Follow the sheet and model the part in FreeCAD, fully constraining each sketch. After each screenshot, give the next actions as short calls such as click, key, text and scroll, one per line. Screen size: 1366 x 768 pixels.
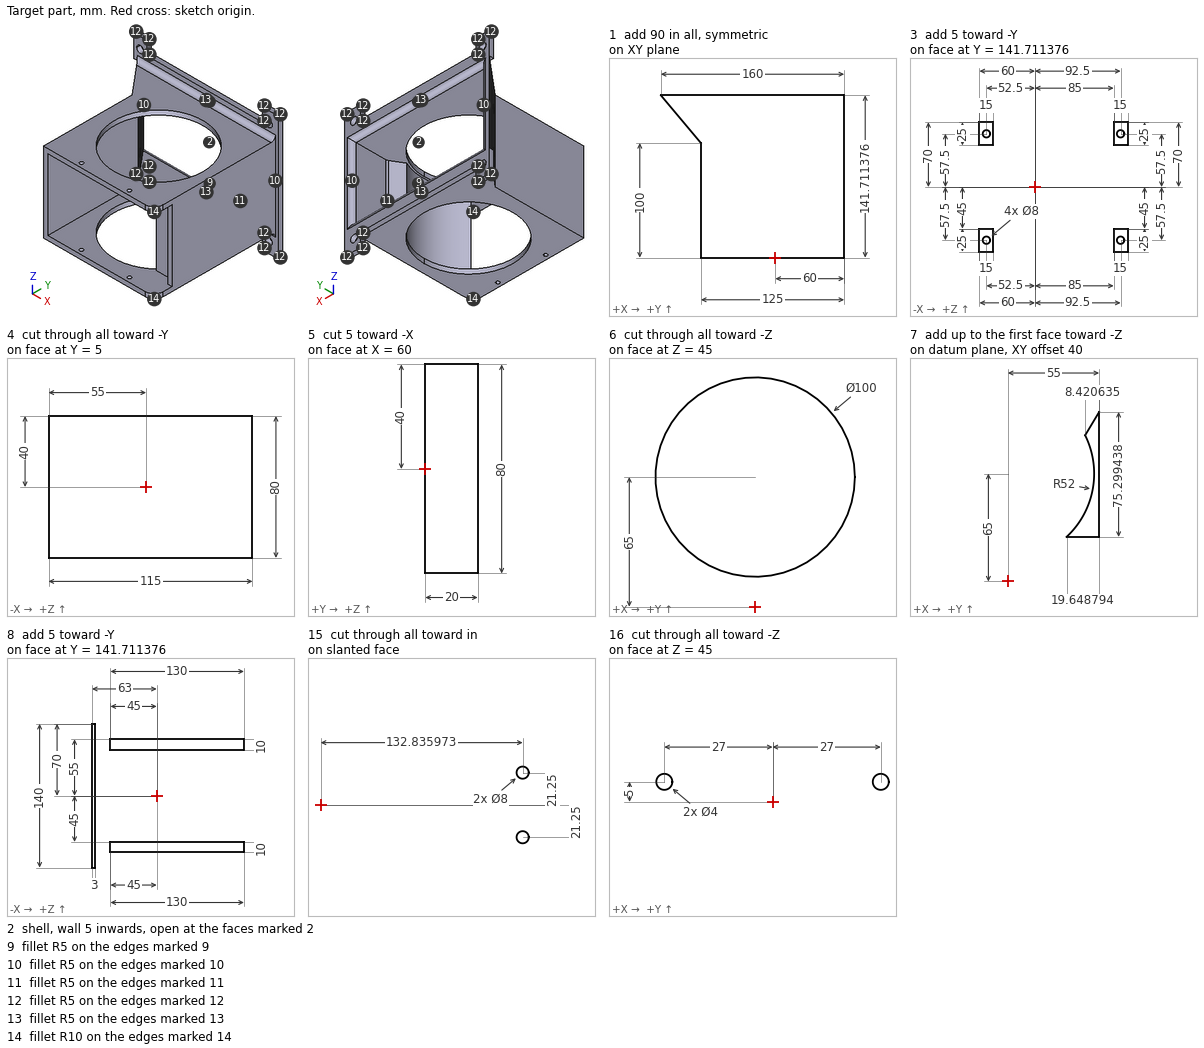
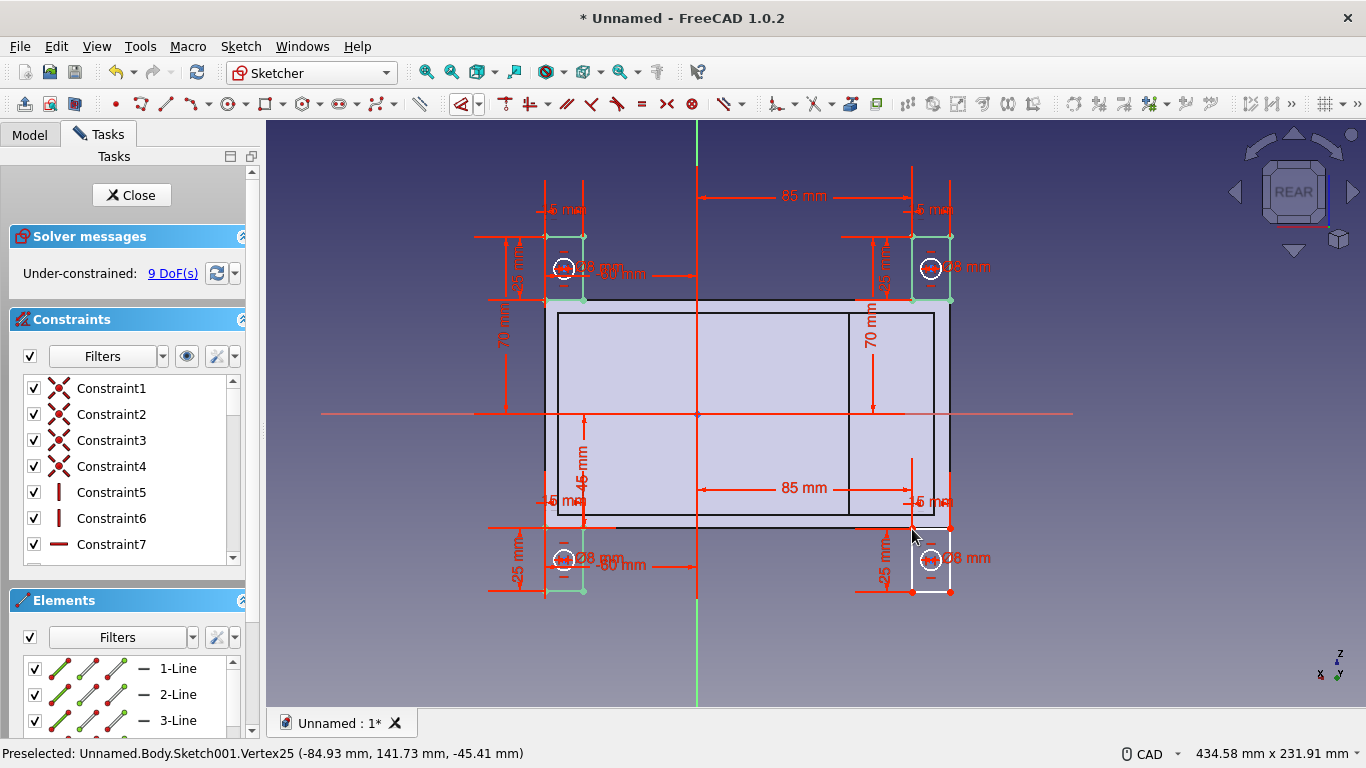
click(912, 529)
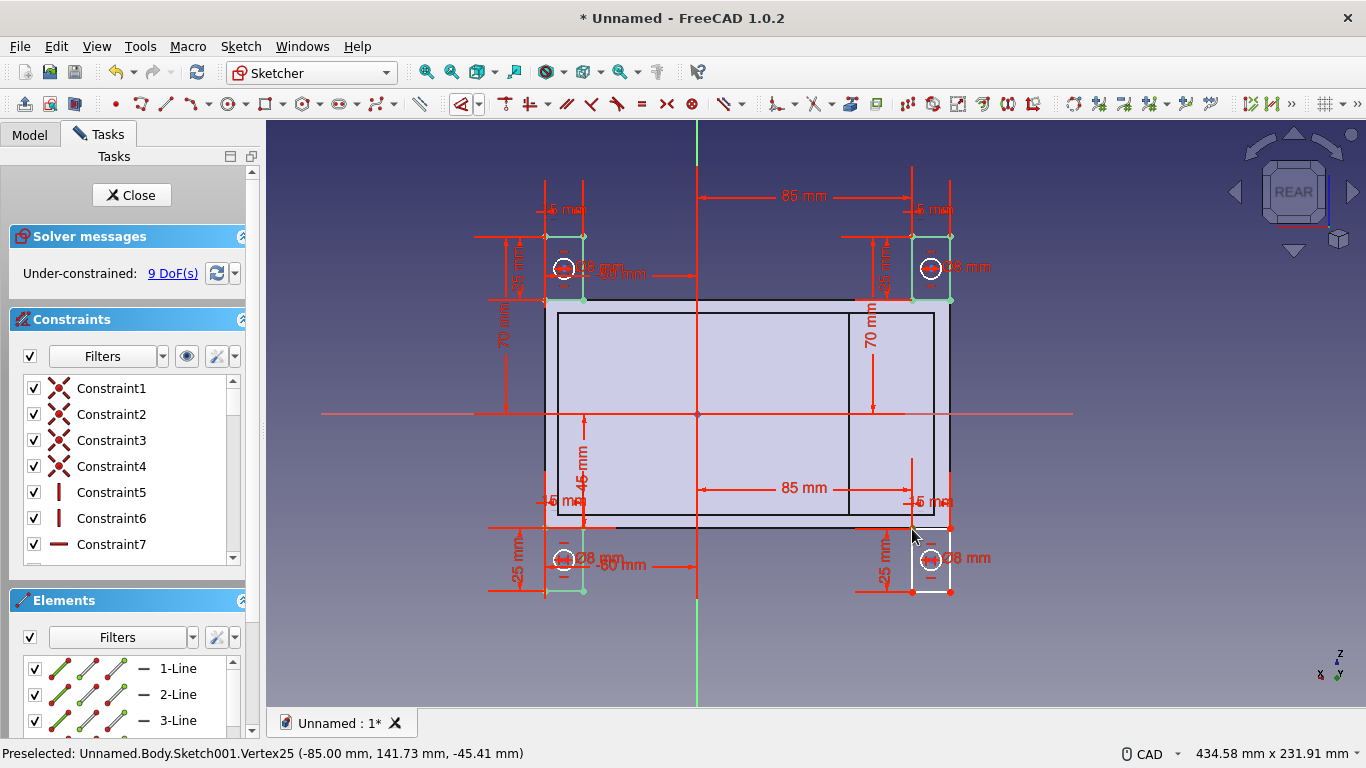
click(478, 104)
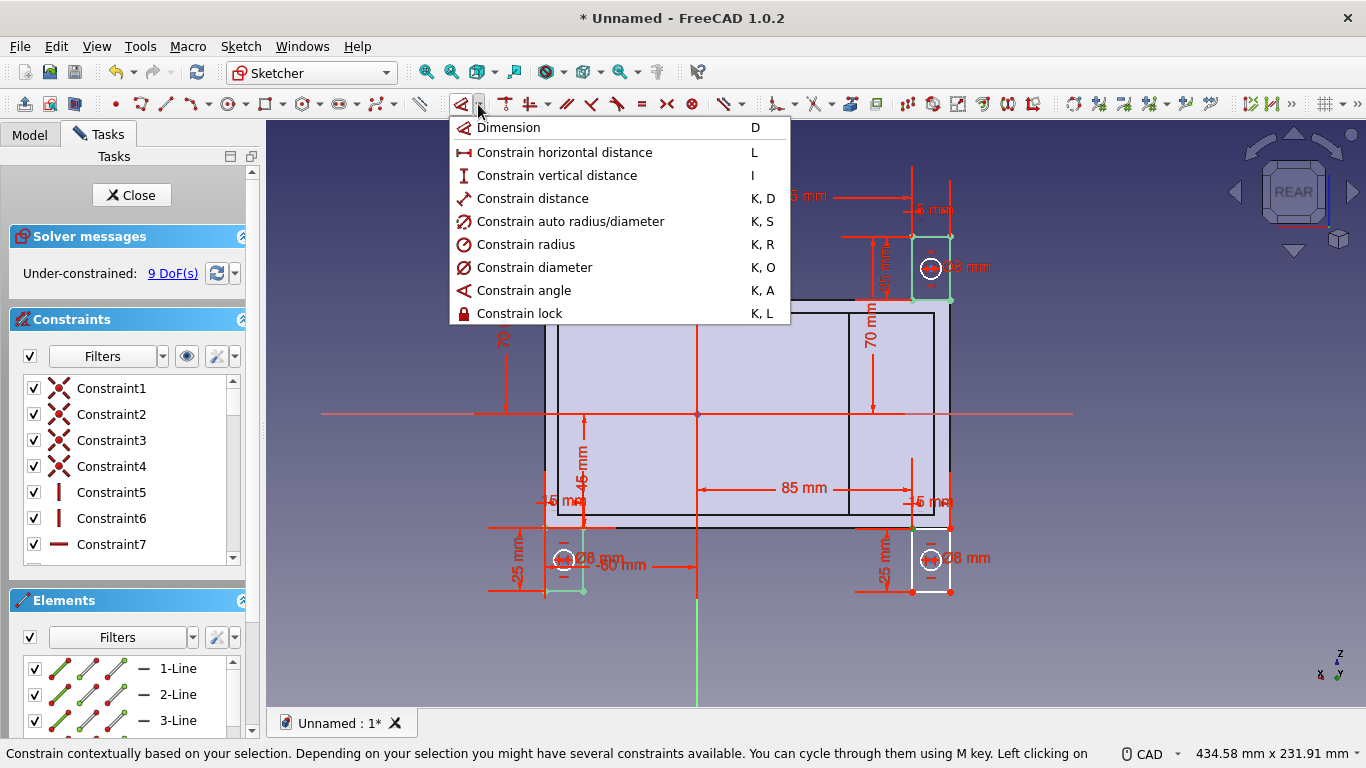
click(620, 176)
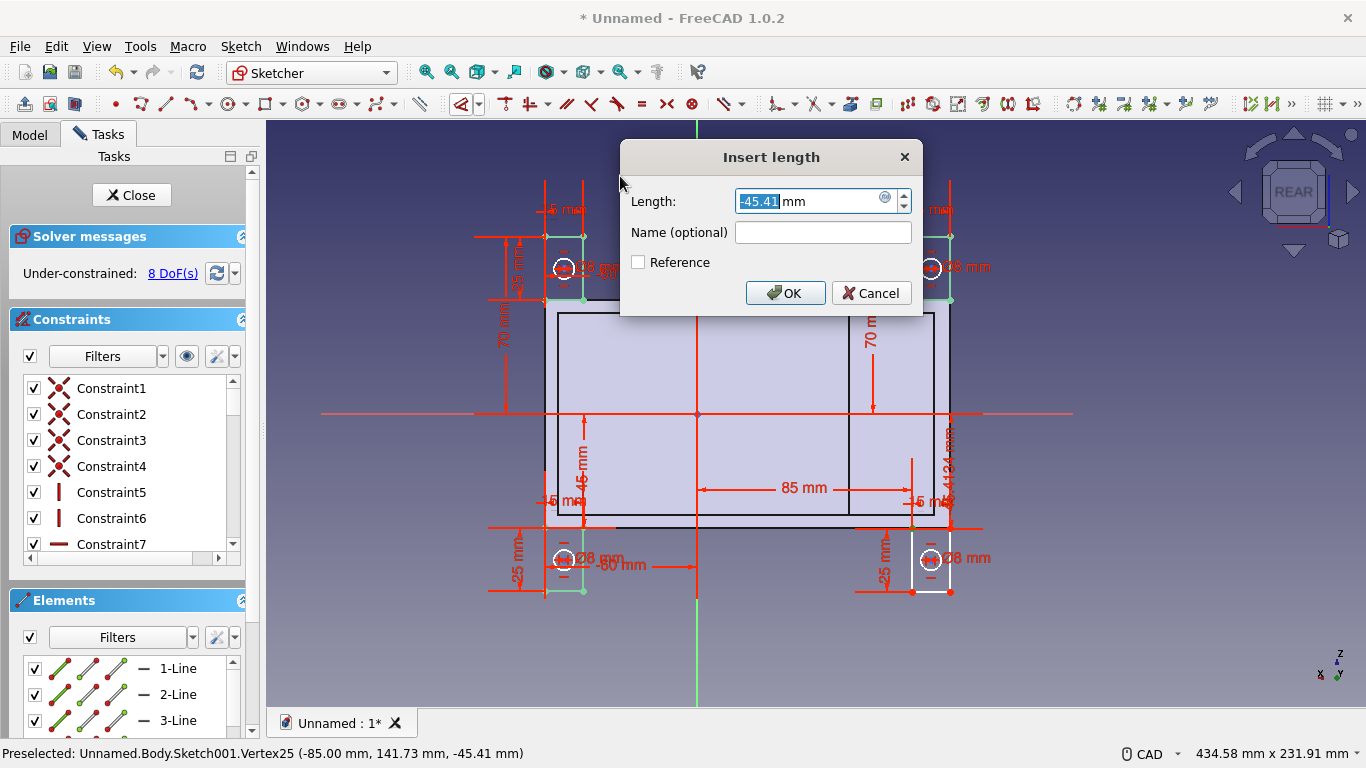
text(-45)
key(Return)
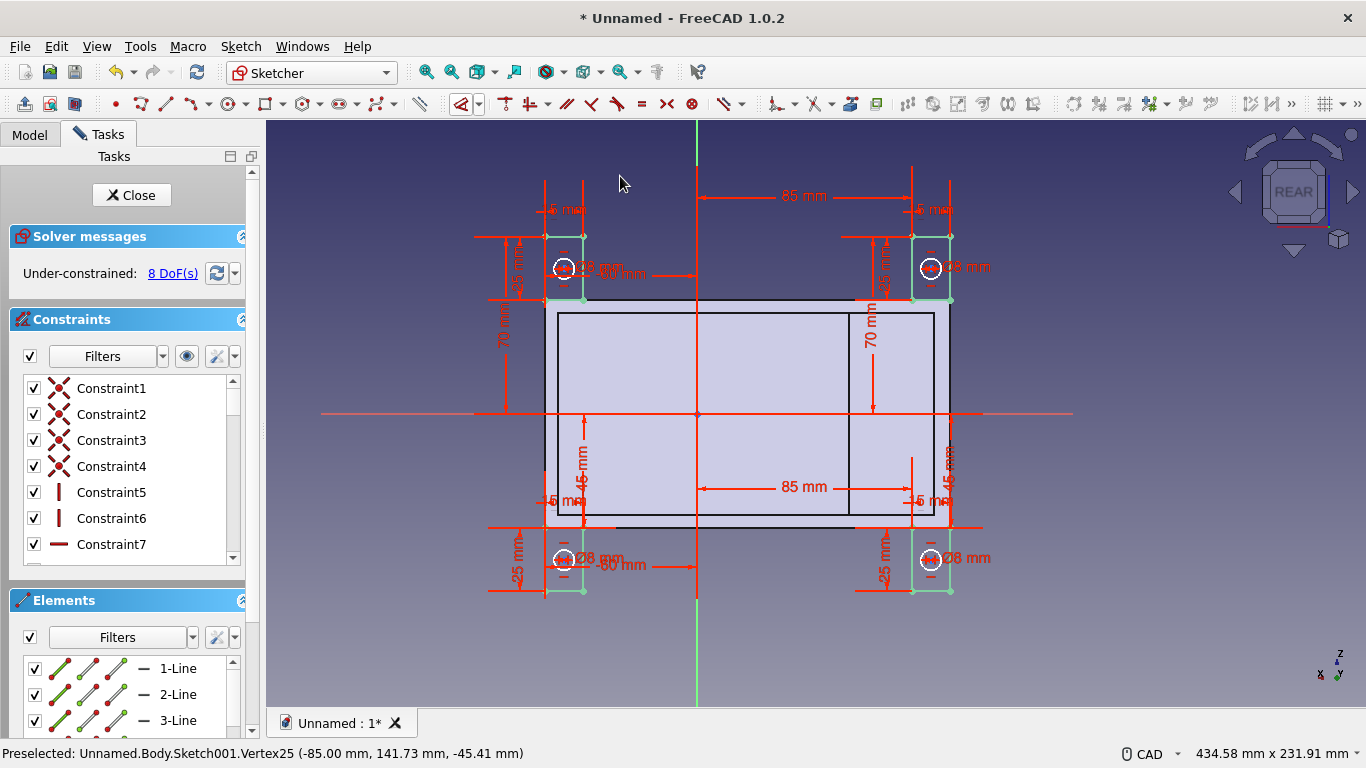
click(564, 560)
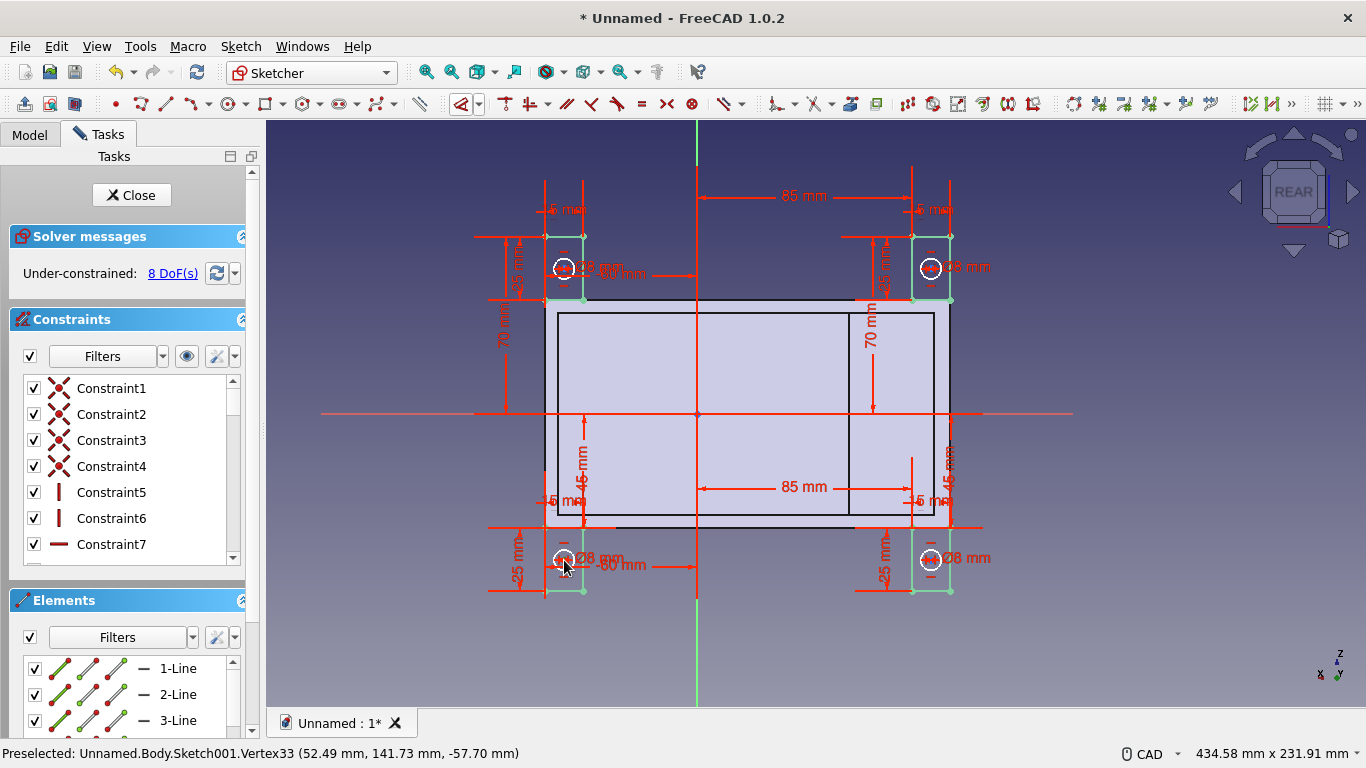
key(l)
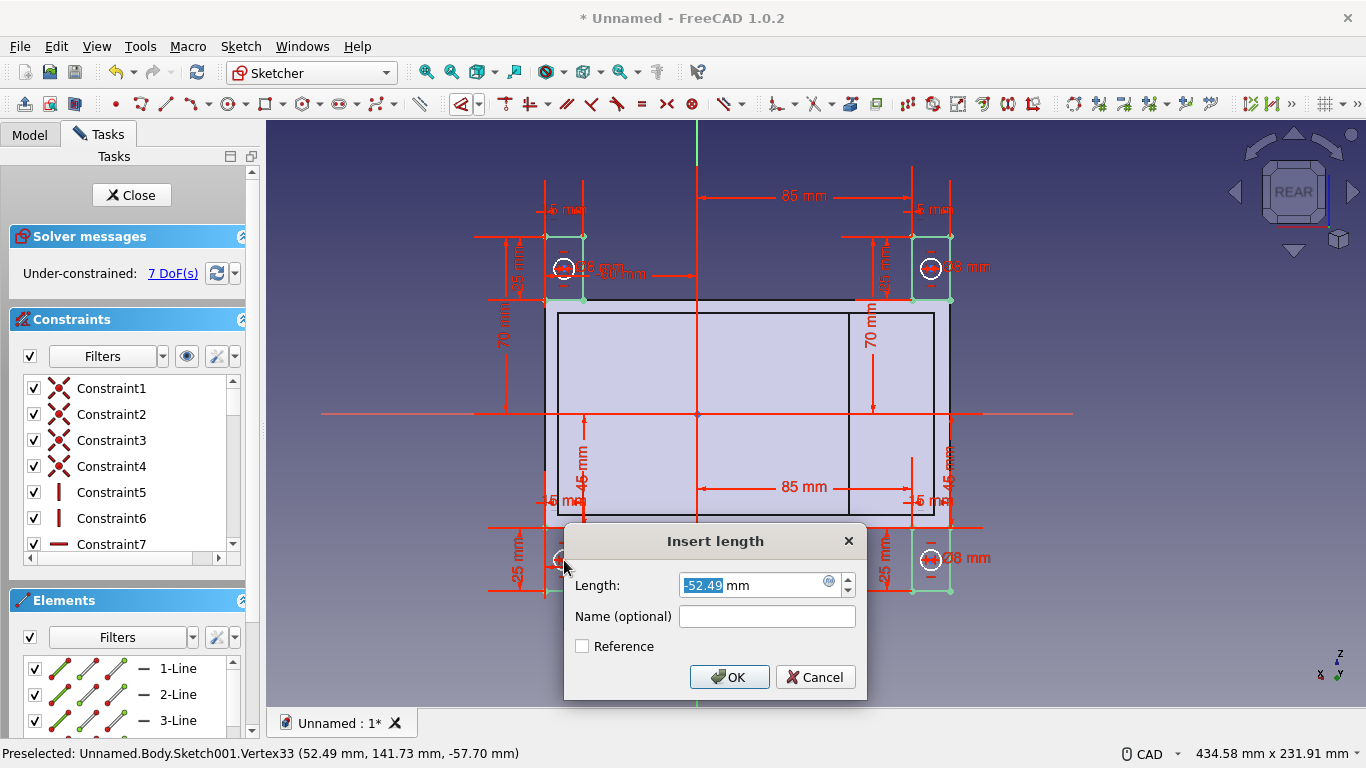
text(-52.5)
key(Return)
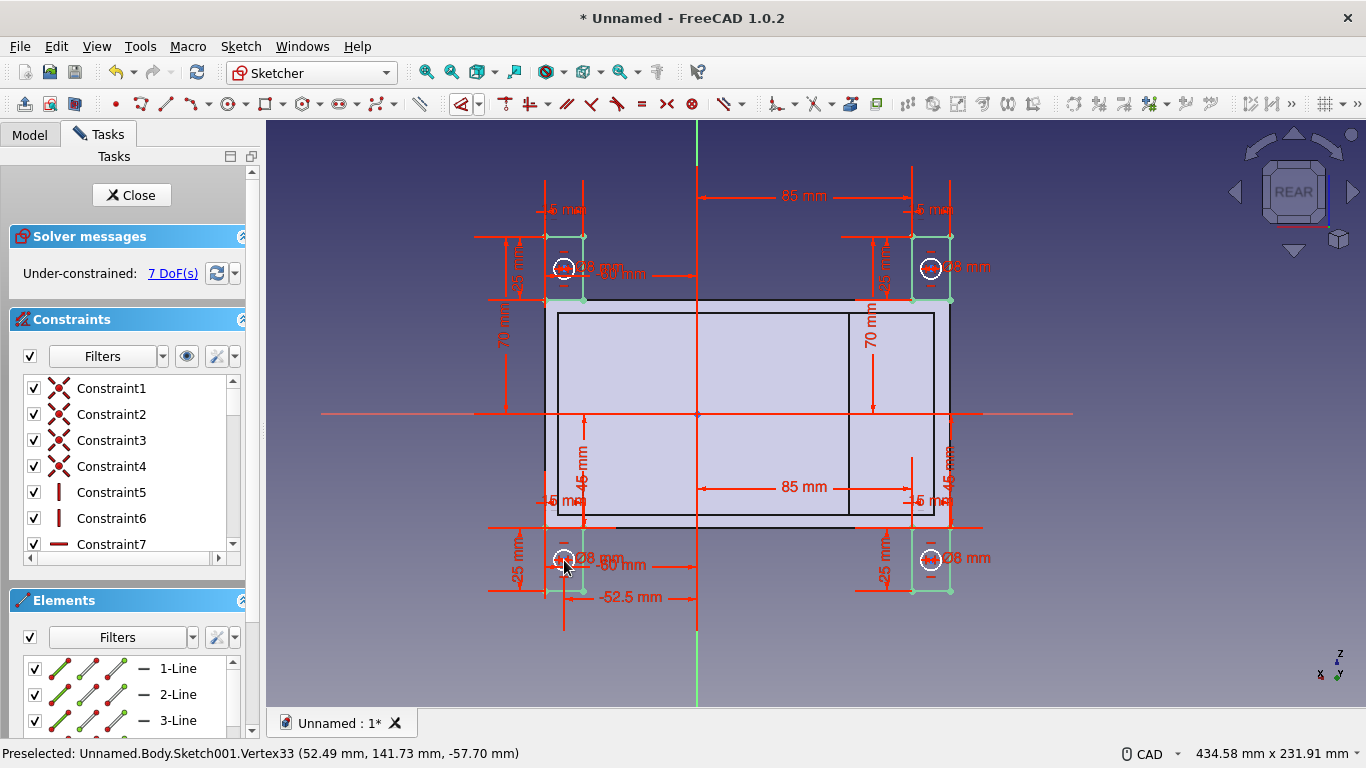
click(564, 560)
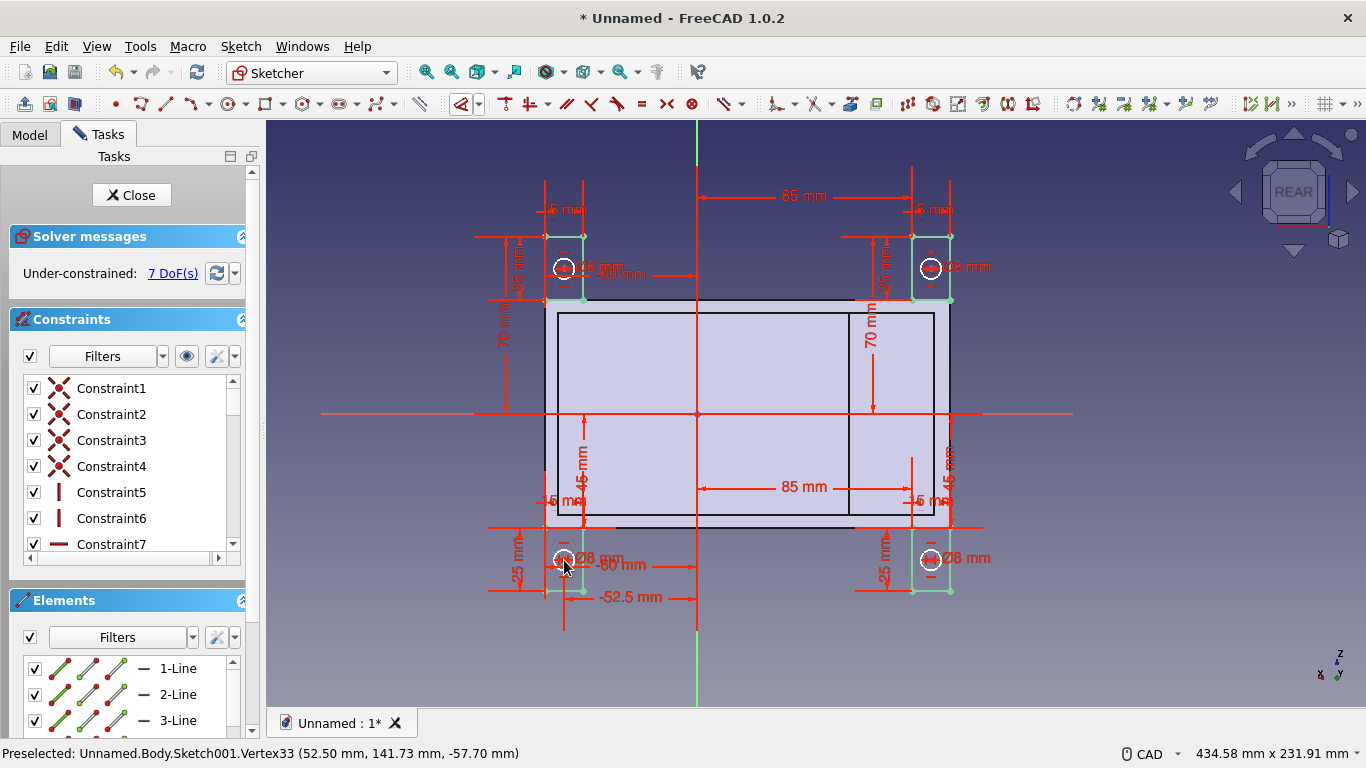
key(i)